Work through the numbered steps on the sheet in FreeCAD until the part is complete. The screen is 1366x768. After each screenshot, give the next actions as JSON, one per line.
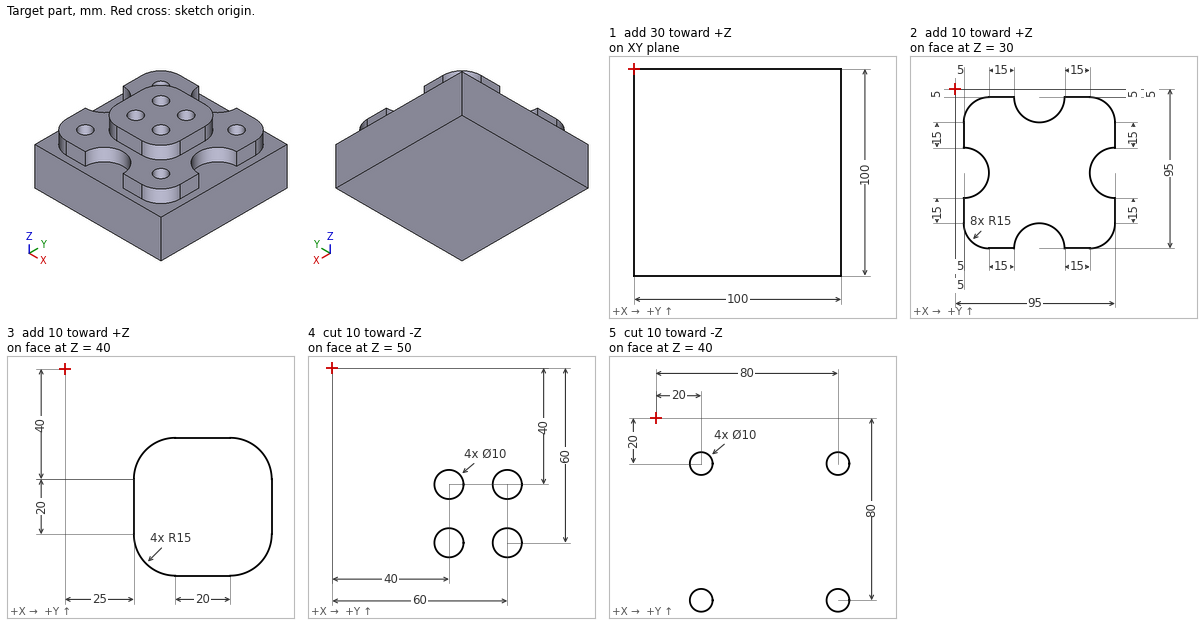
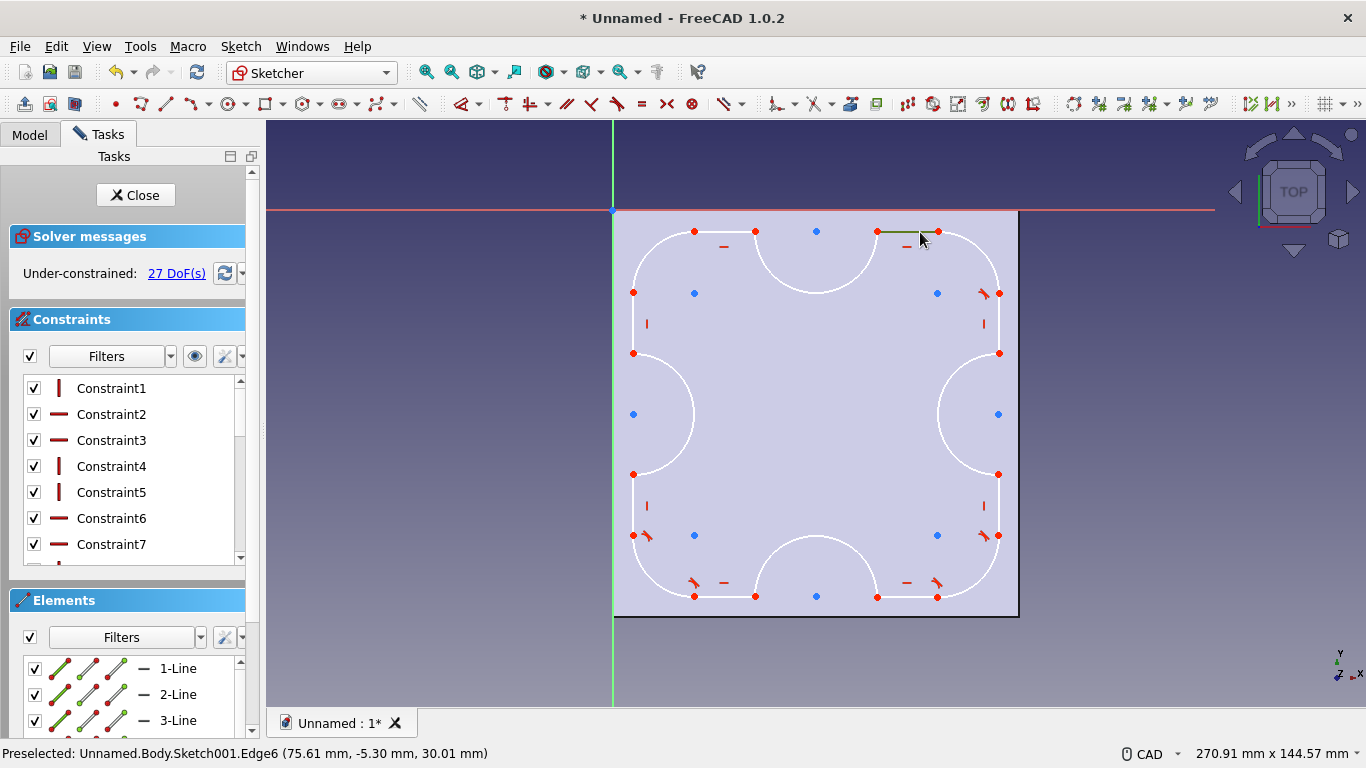
{"action": "left_click", "coordinate": [992, 266]}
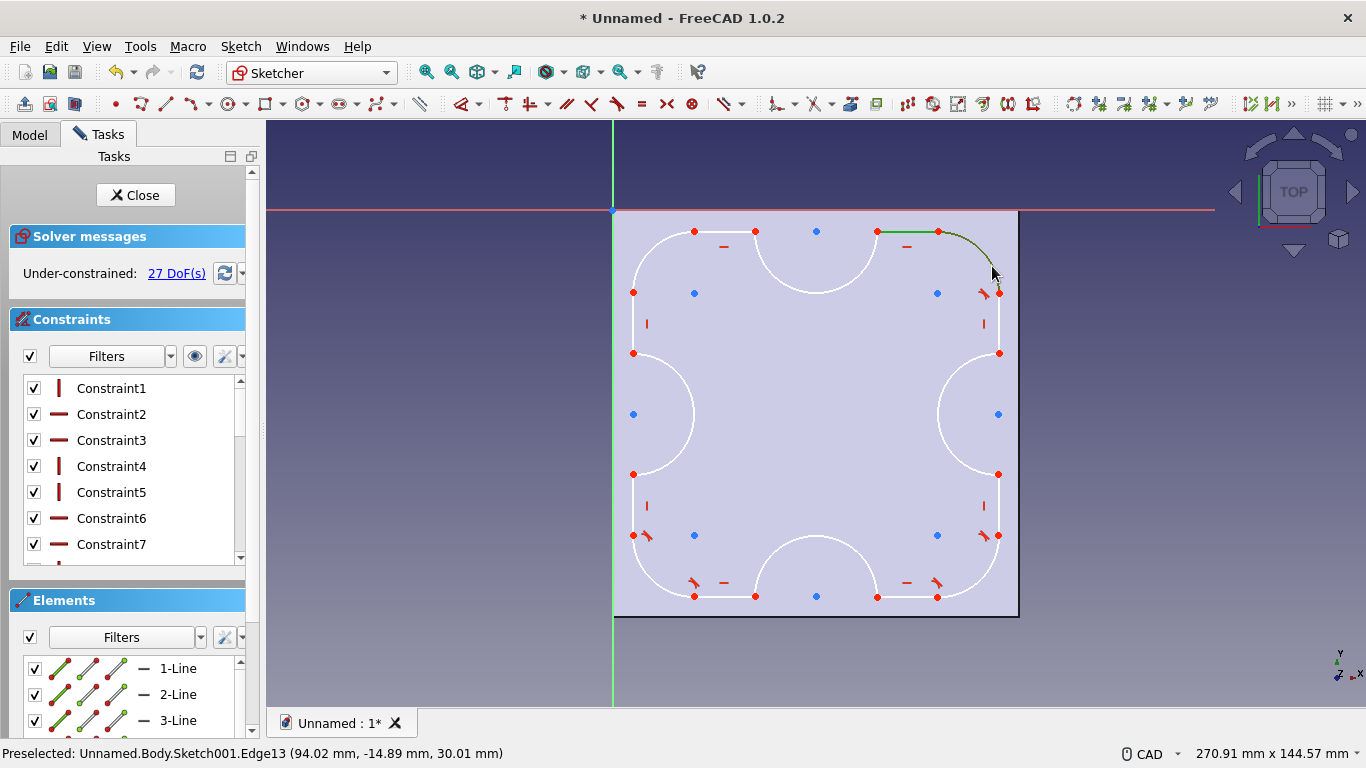
{"action": "left_click", "coordinate": [617, 104]}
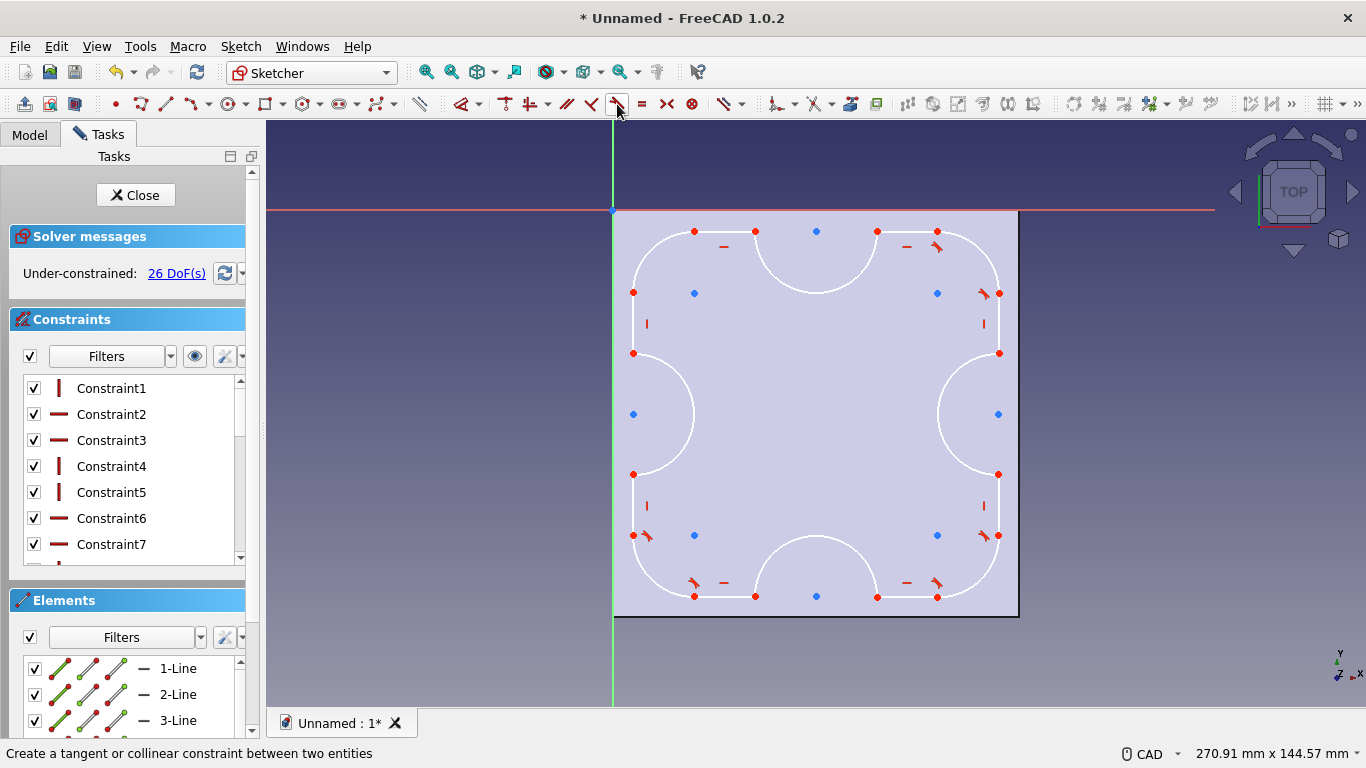
{"action": "left_click", "coordinate": [737, 232]}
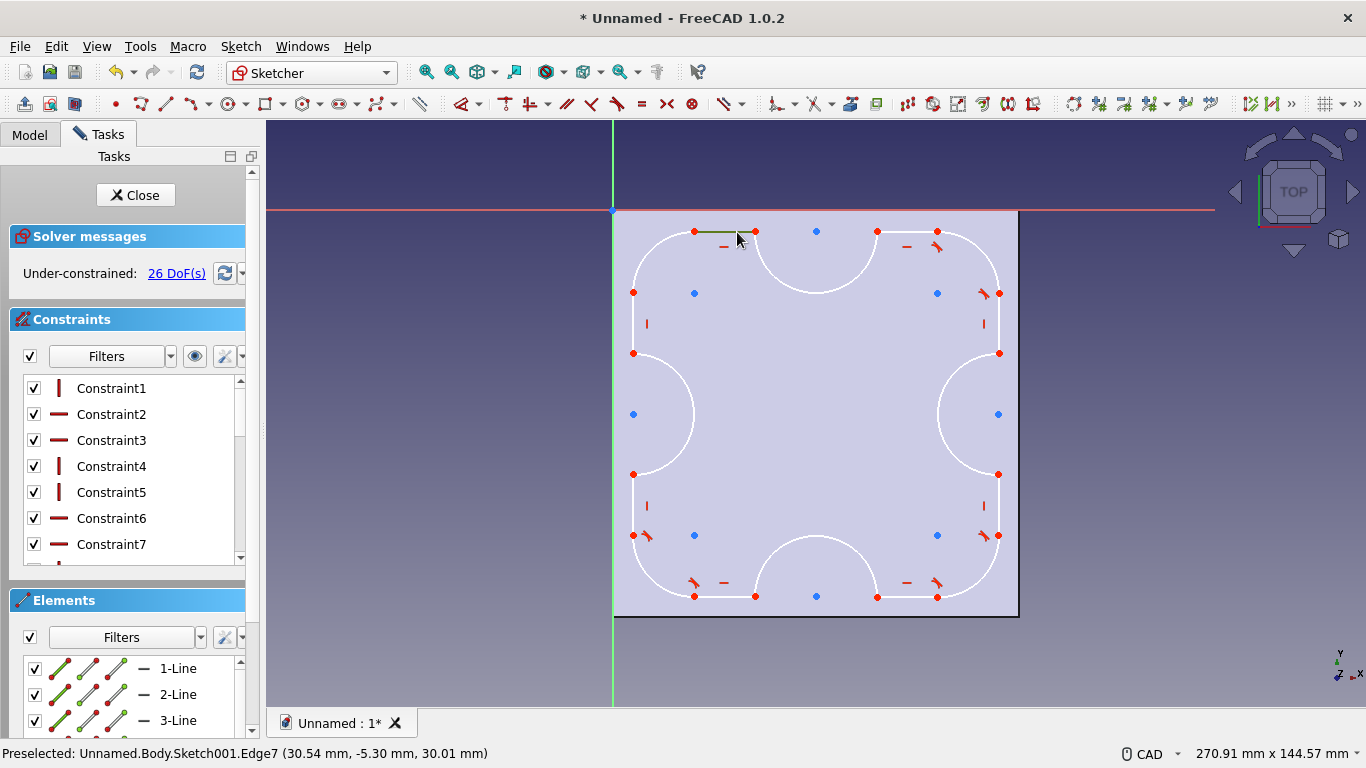
{"action": "left_click", "coordinate": [666, 239]}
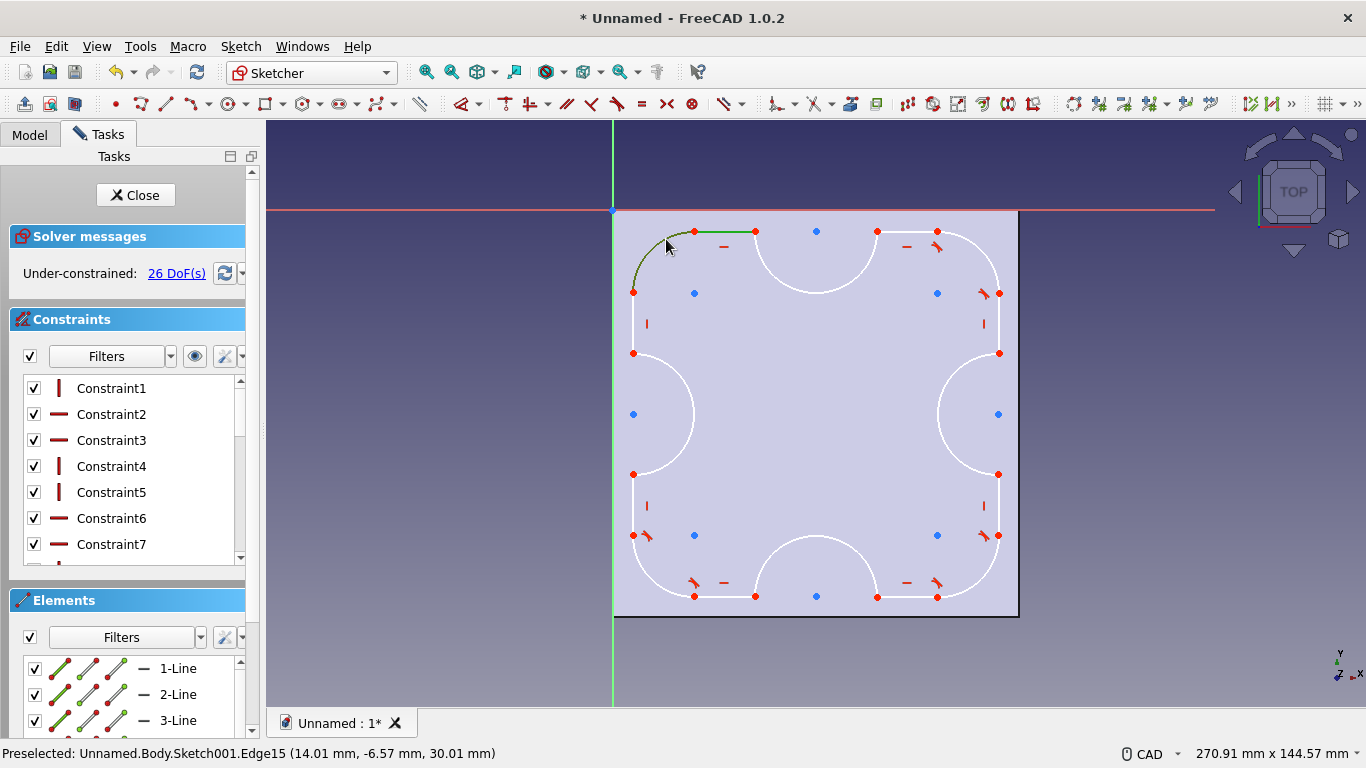
{"action": "left_click", "coordinate": [617, 104]}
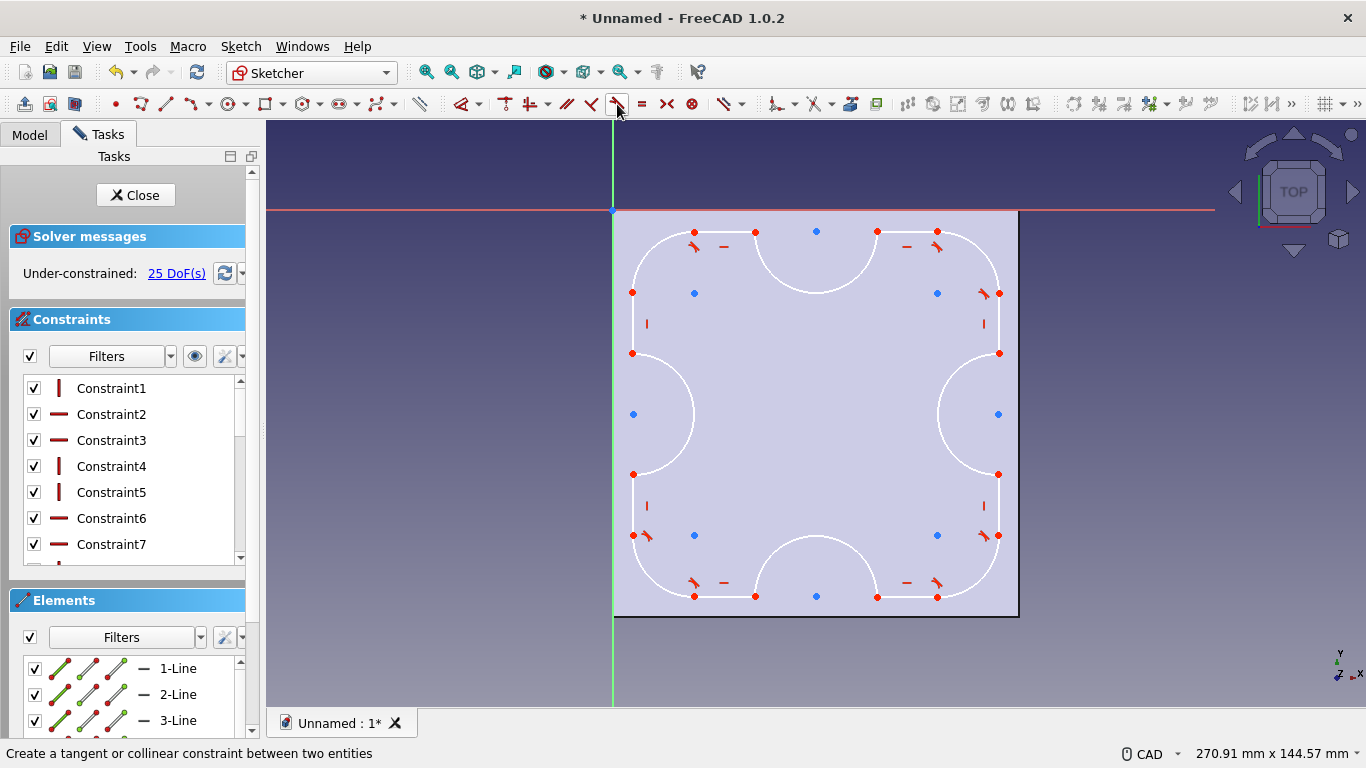
{"action": "left_click", "coordinate": [633, 311]}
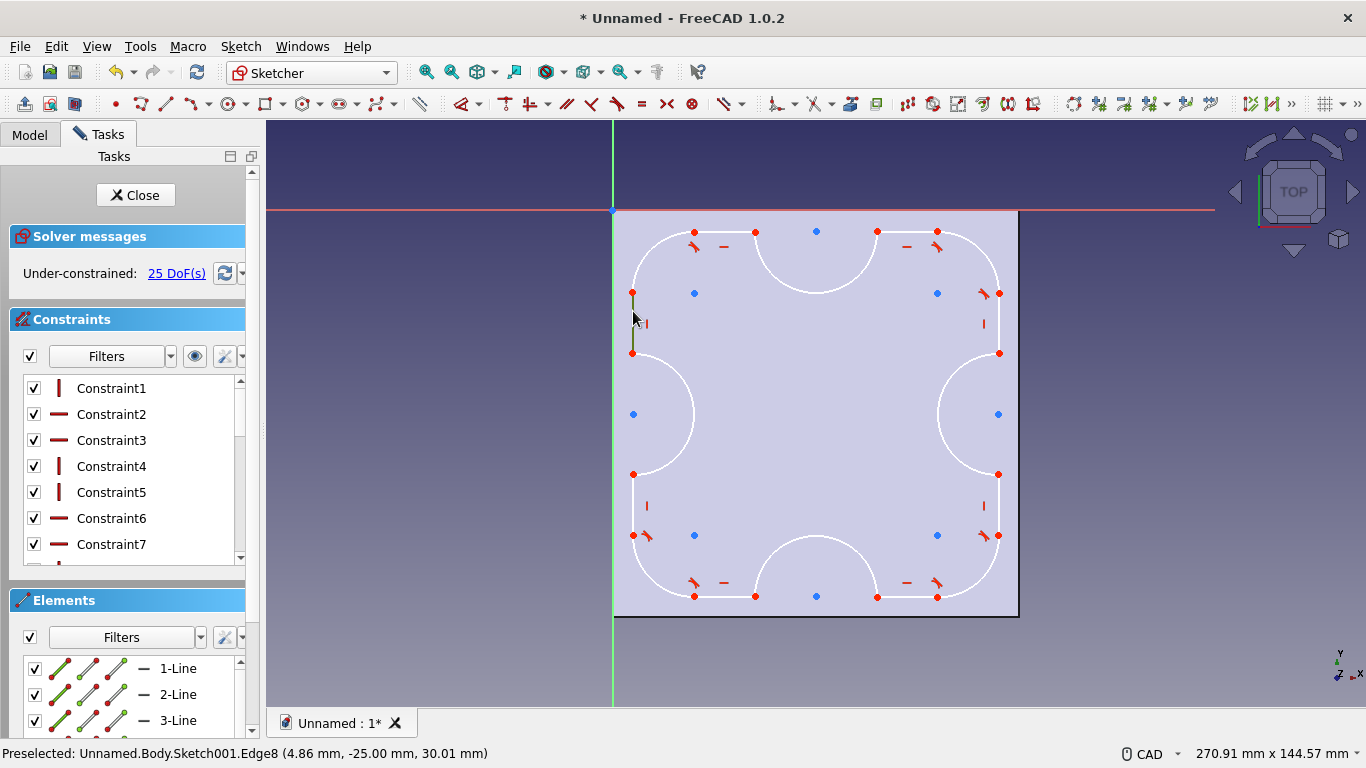
{"action": "left_click", "coordinate": [666, 239]}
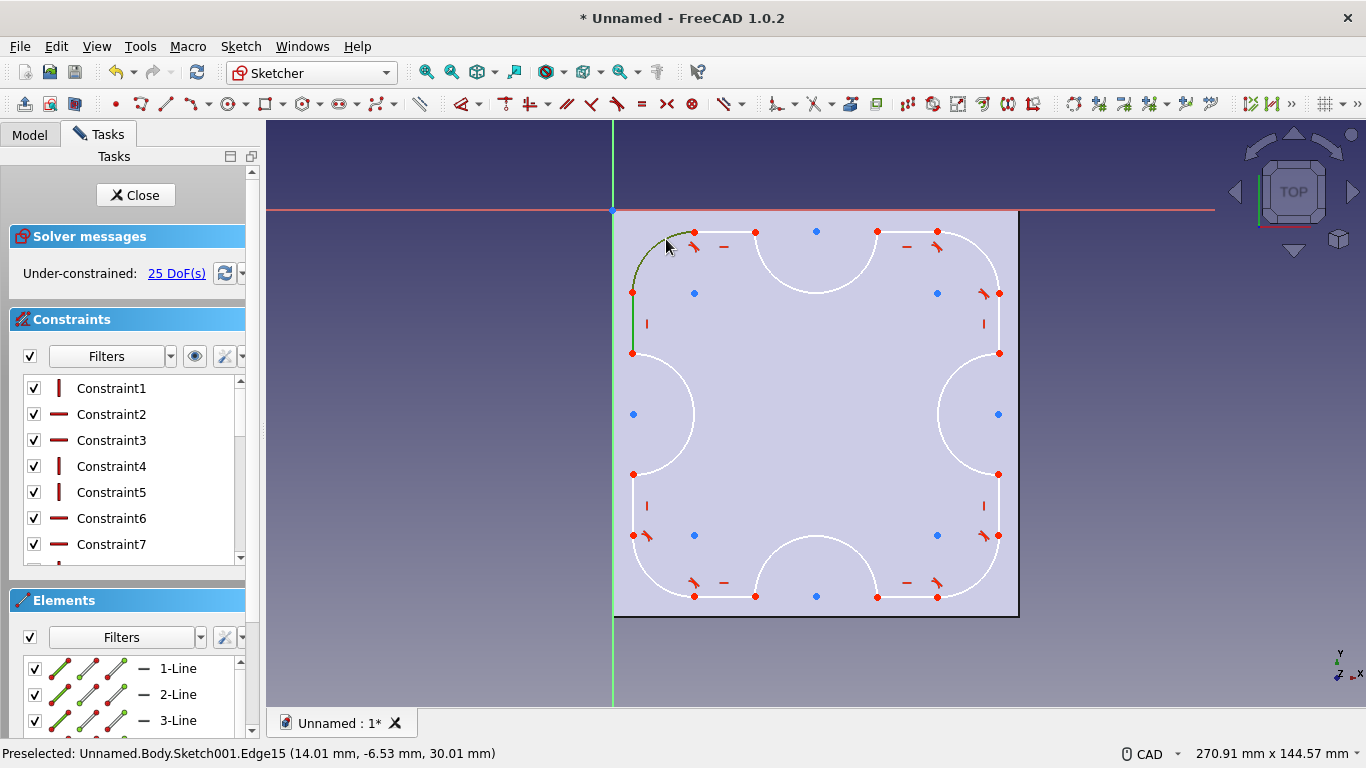
{"action": "left_click", "coordinate": [617, 104]}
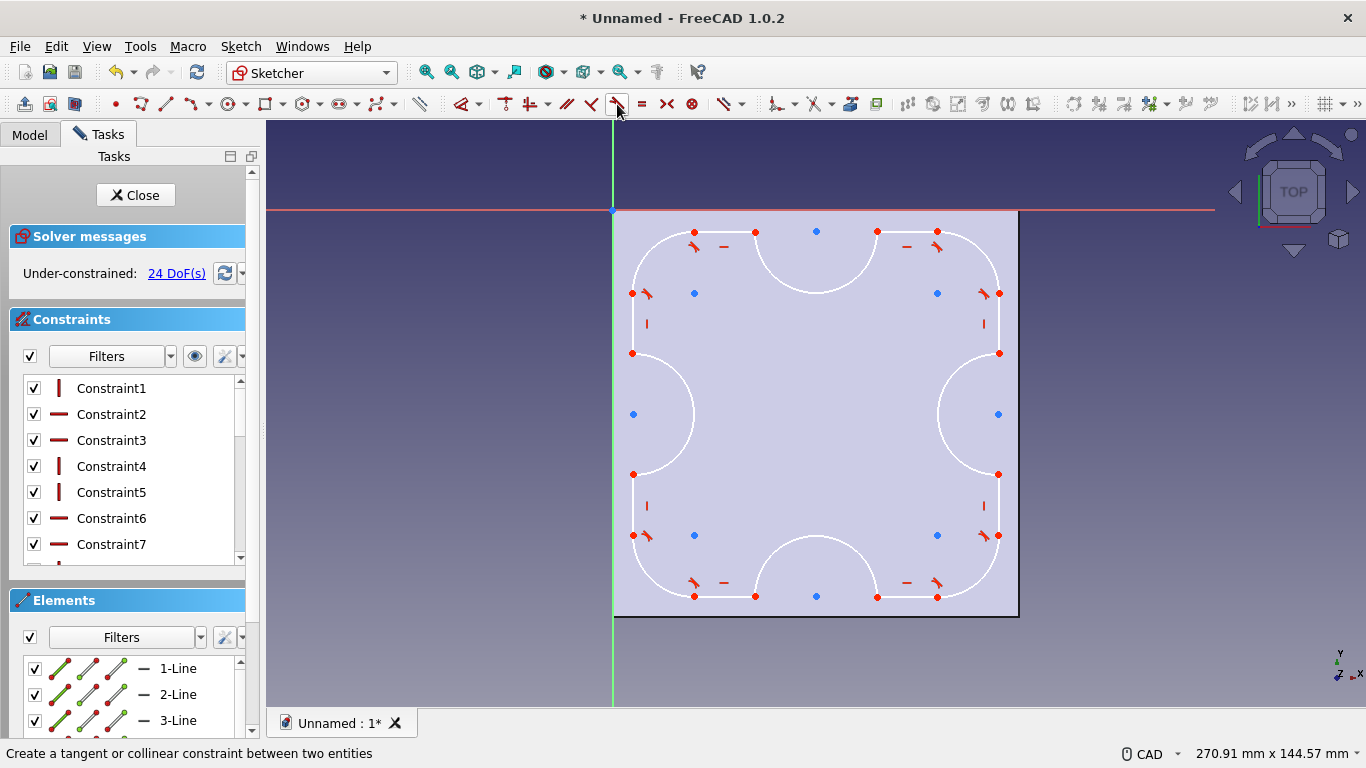
{"action": "left_click", "coordinate": [640, 563]}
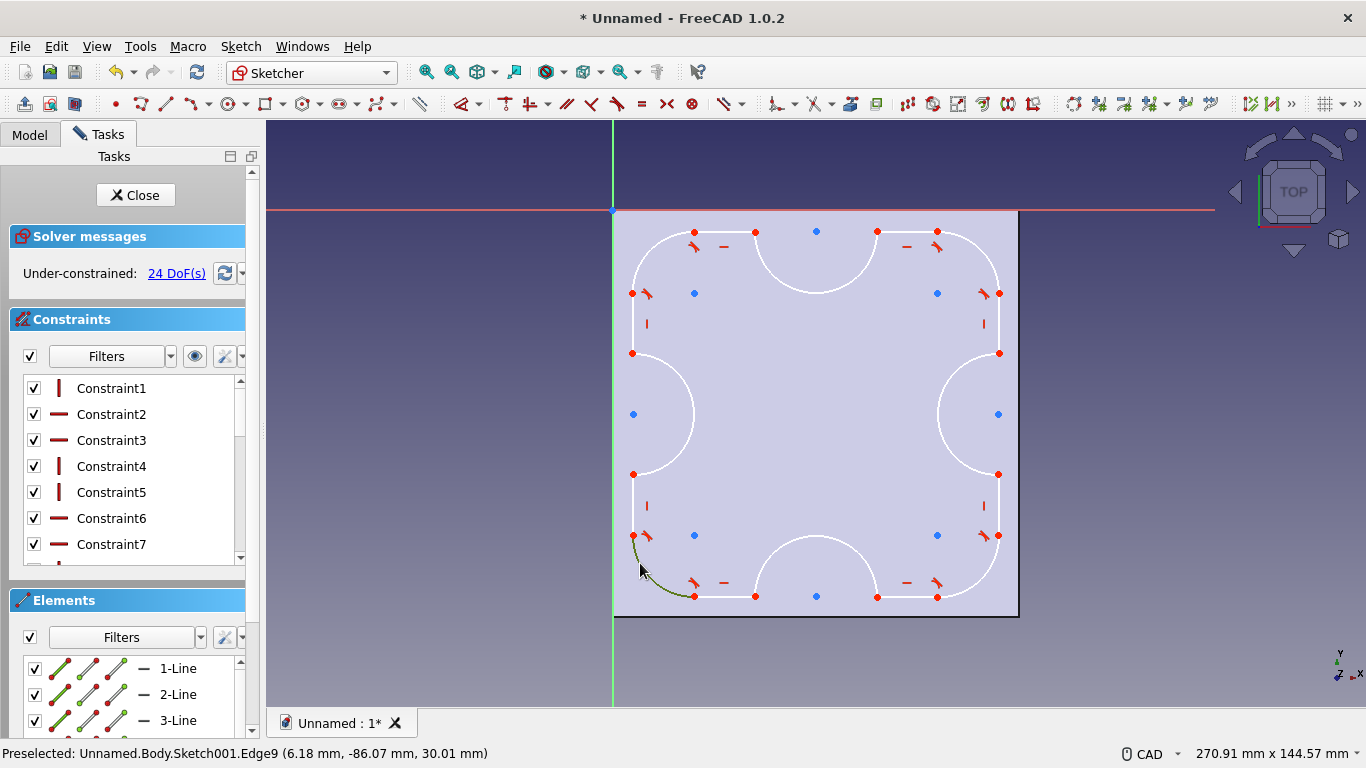
{"action": "left_click", "coordinate": [852, 548]}